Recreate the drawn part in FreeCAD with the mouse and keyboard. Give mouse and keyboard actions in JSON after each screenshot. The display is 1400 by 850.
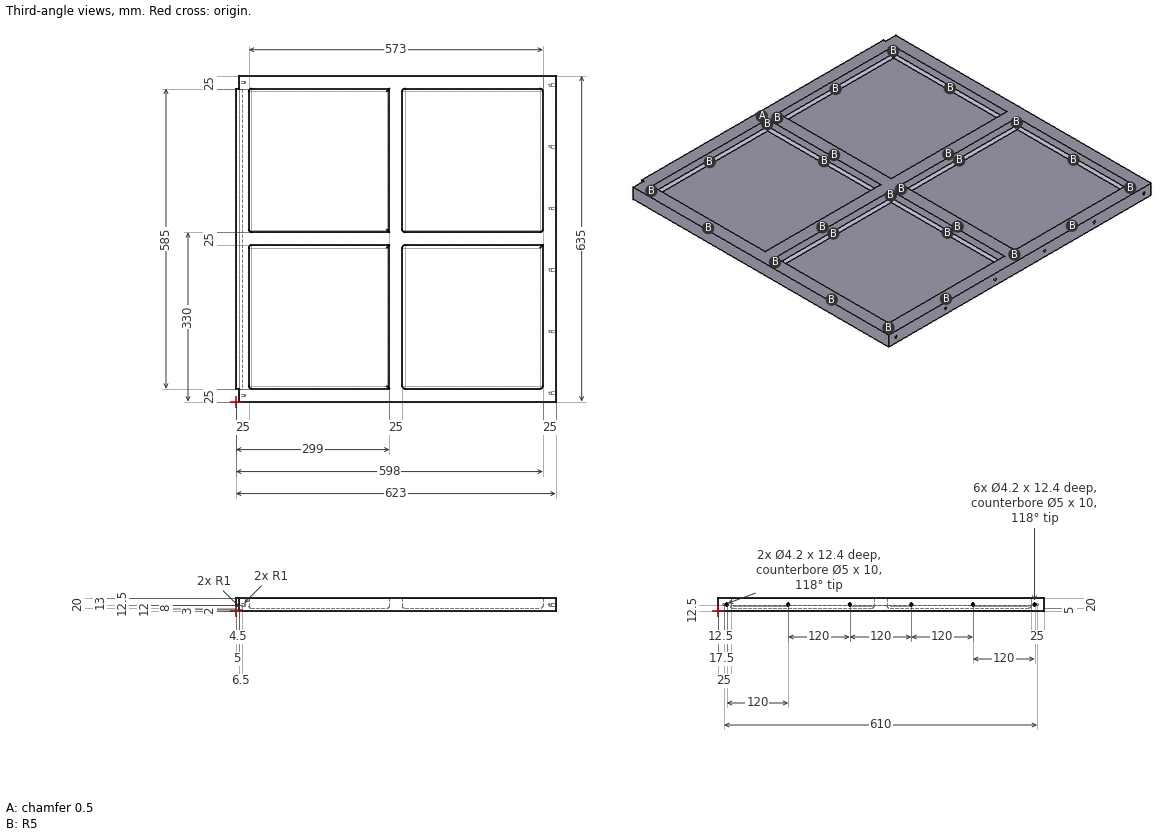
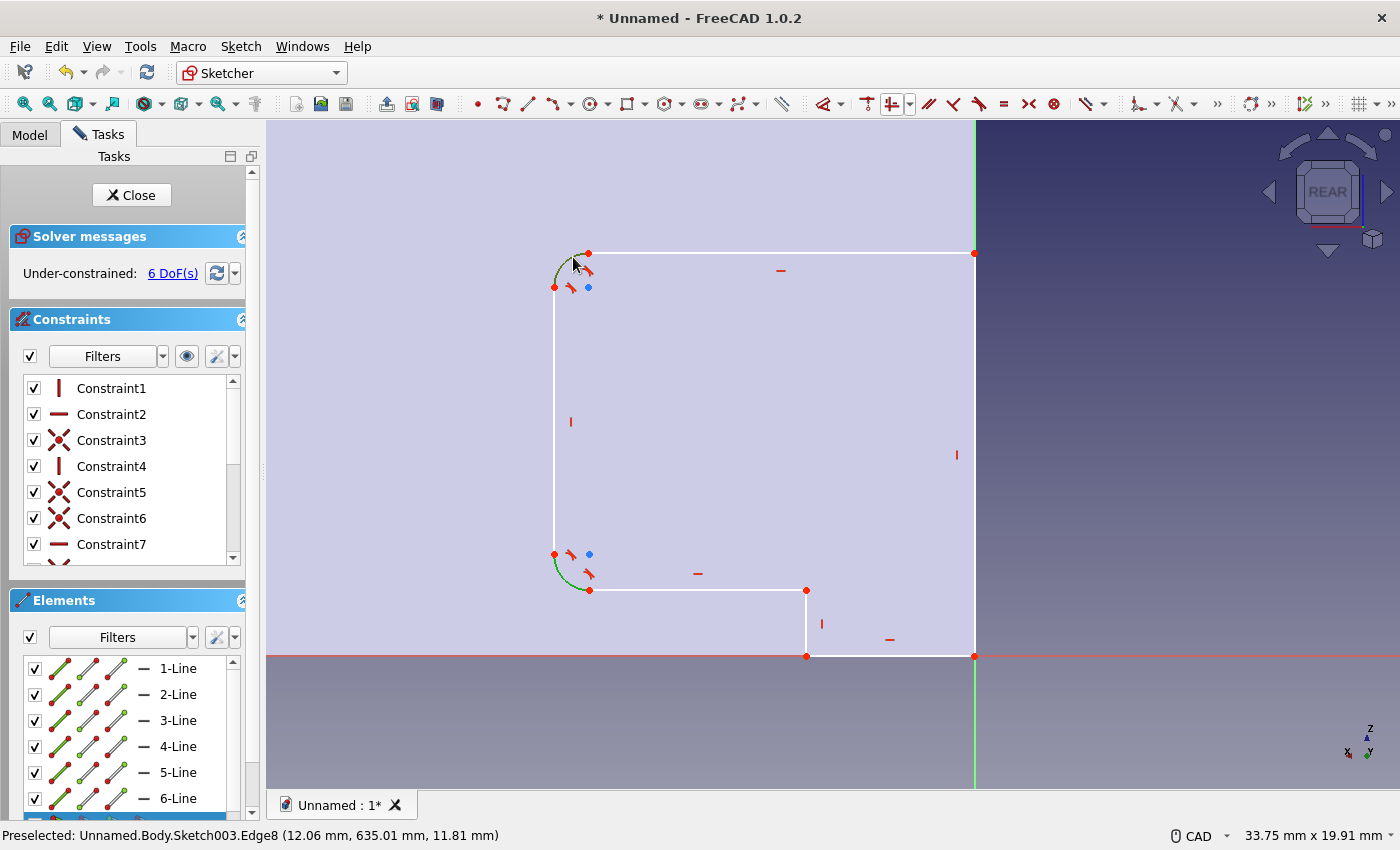
{"action": "left_click", "coordinate": [1004, 104]}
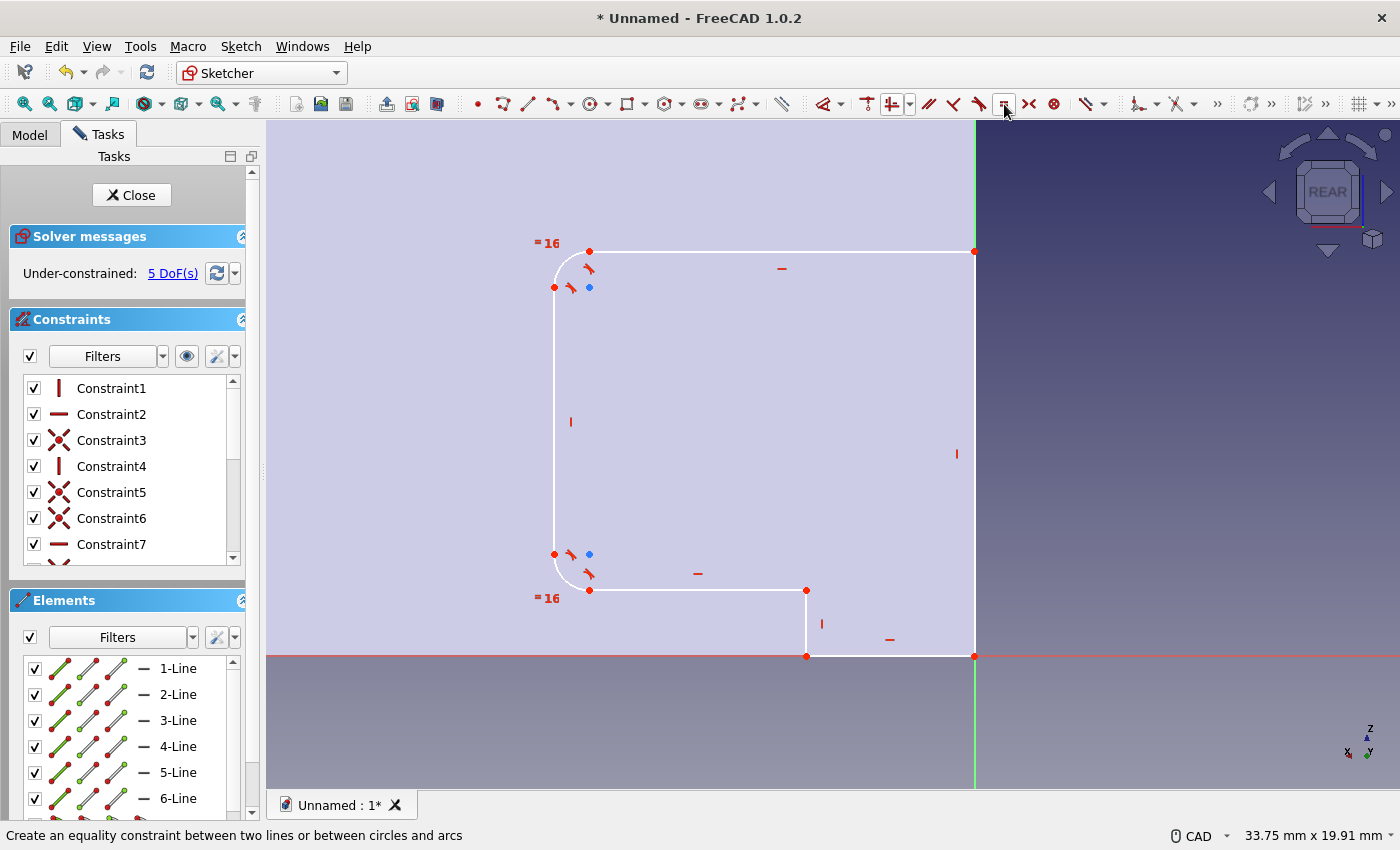
{"action": "left_click", "coordinate": [822, 104]}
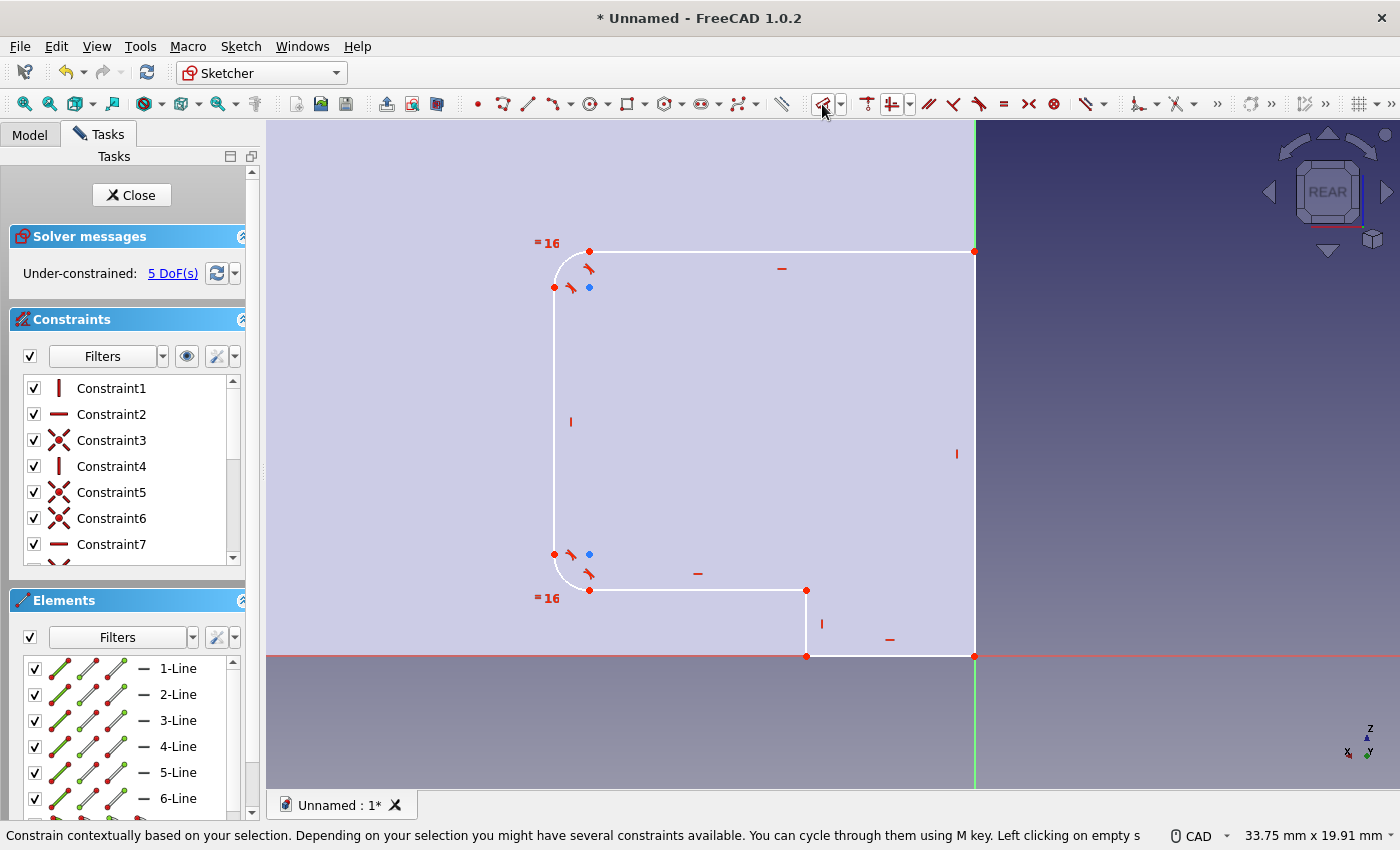
{"action": "left_click", "coordinate": [558, 571]}
{"action": "left_click", "coordinate": [529, 586]}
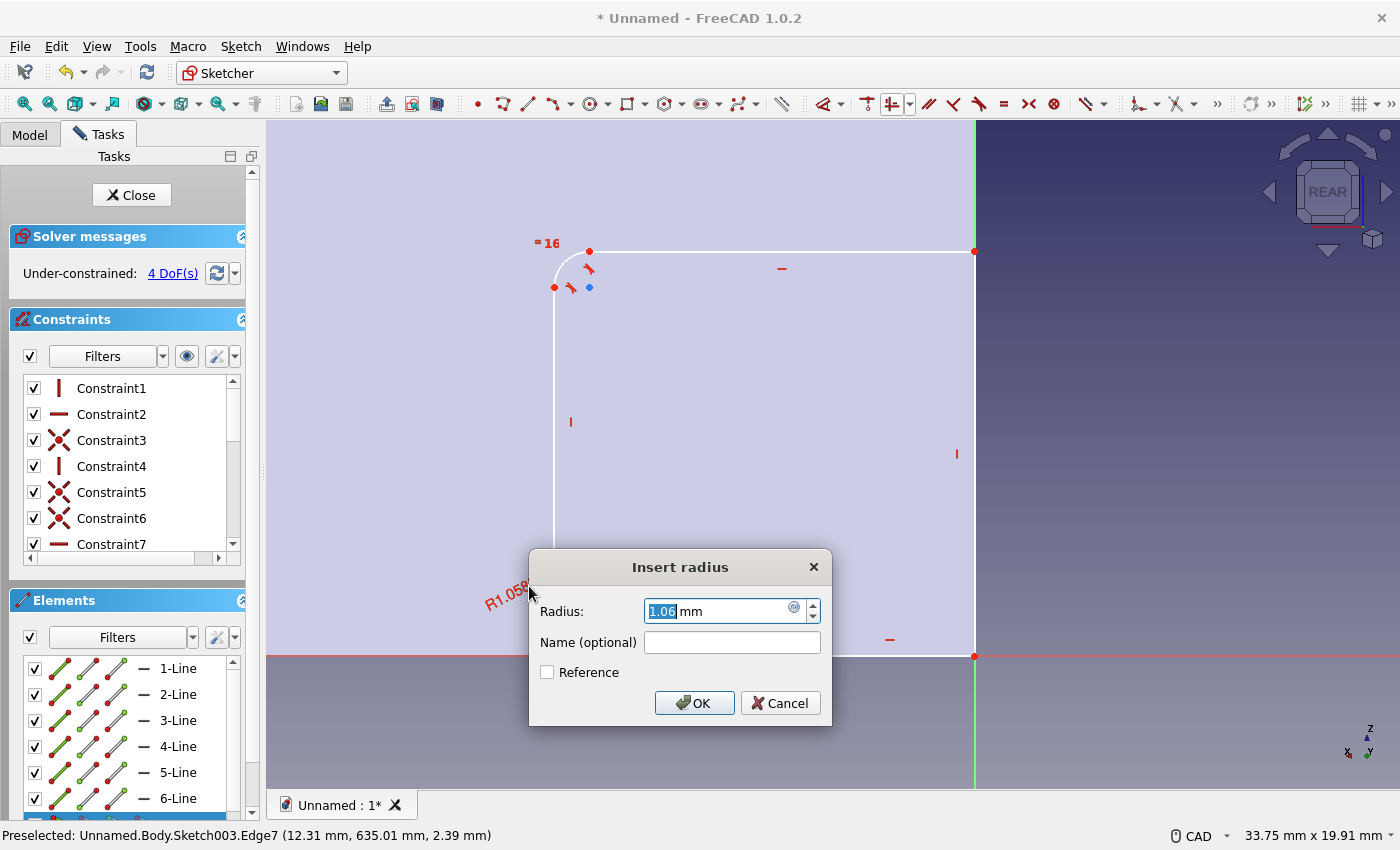
{"action": "type", "text": "1"}
{"action": "key", "text": "Return"}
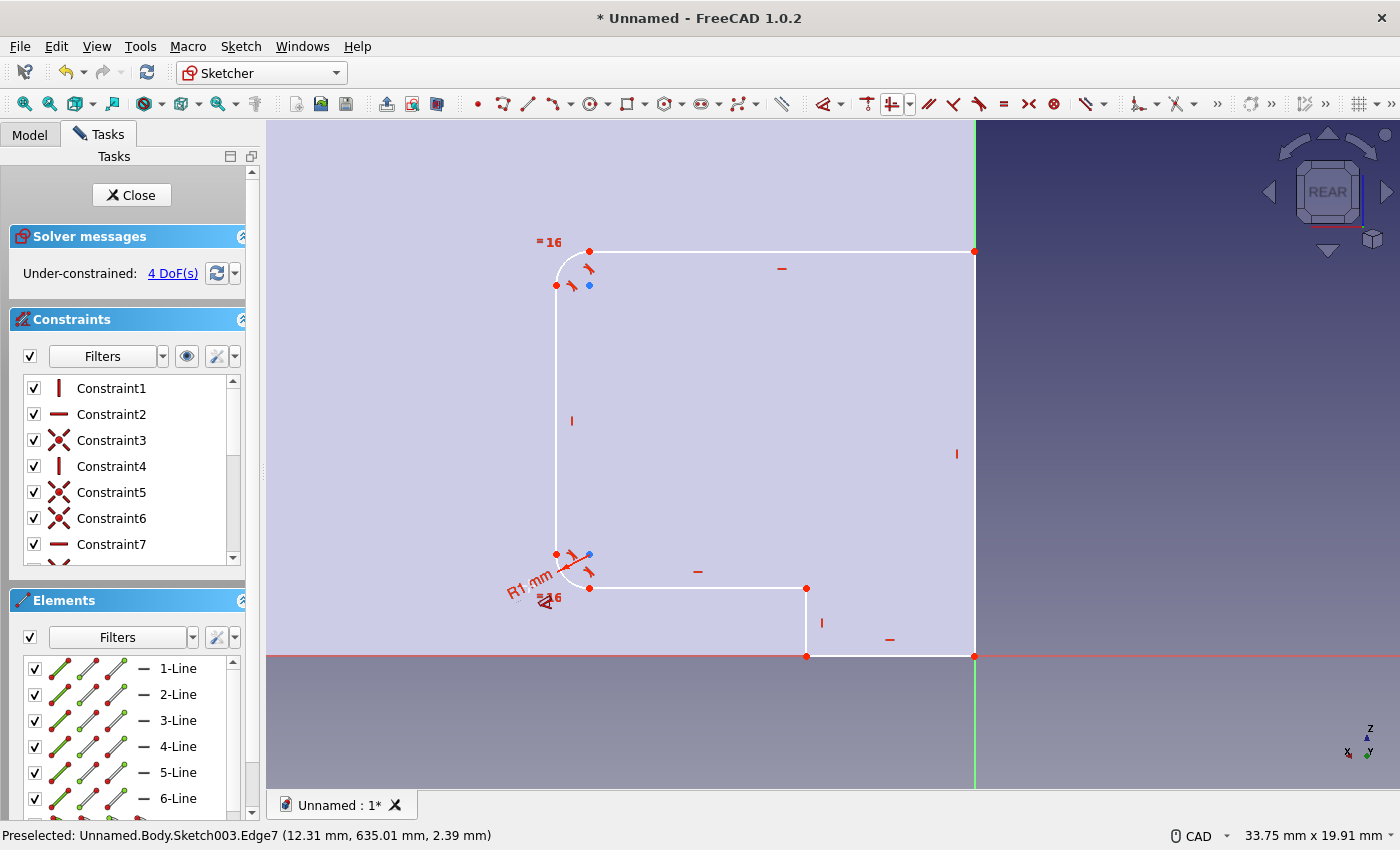
{"action": "left_click", "coordinate": [556, 366]}
{"action": "left_click", "coordinate": [522, 420]}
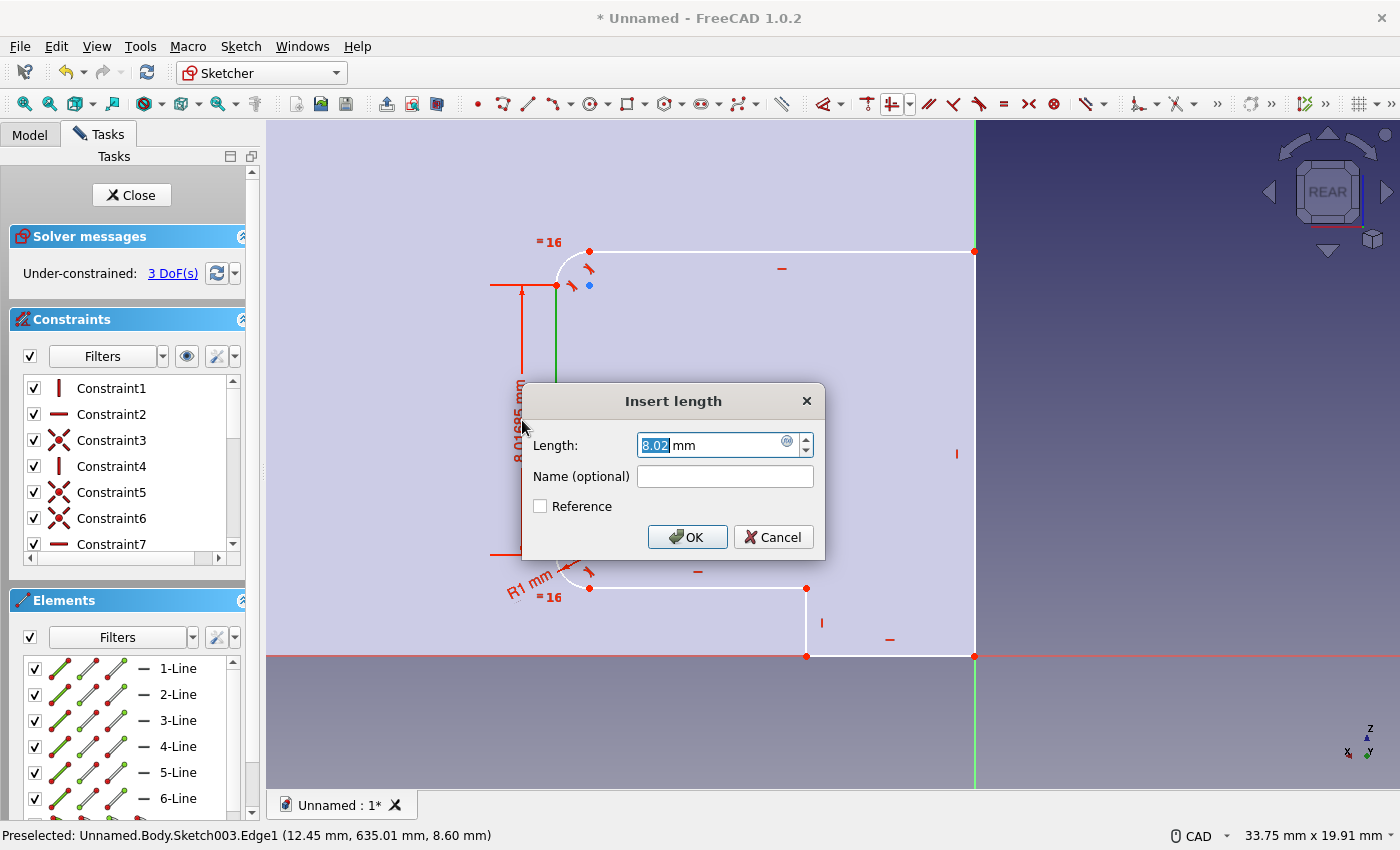
{"action": "type", "text": "8"}
{"action": "key", "text": "Return"}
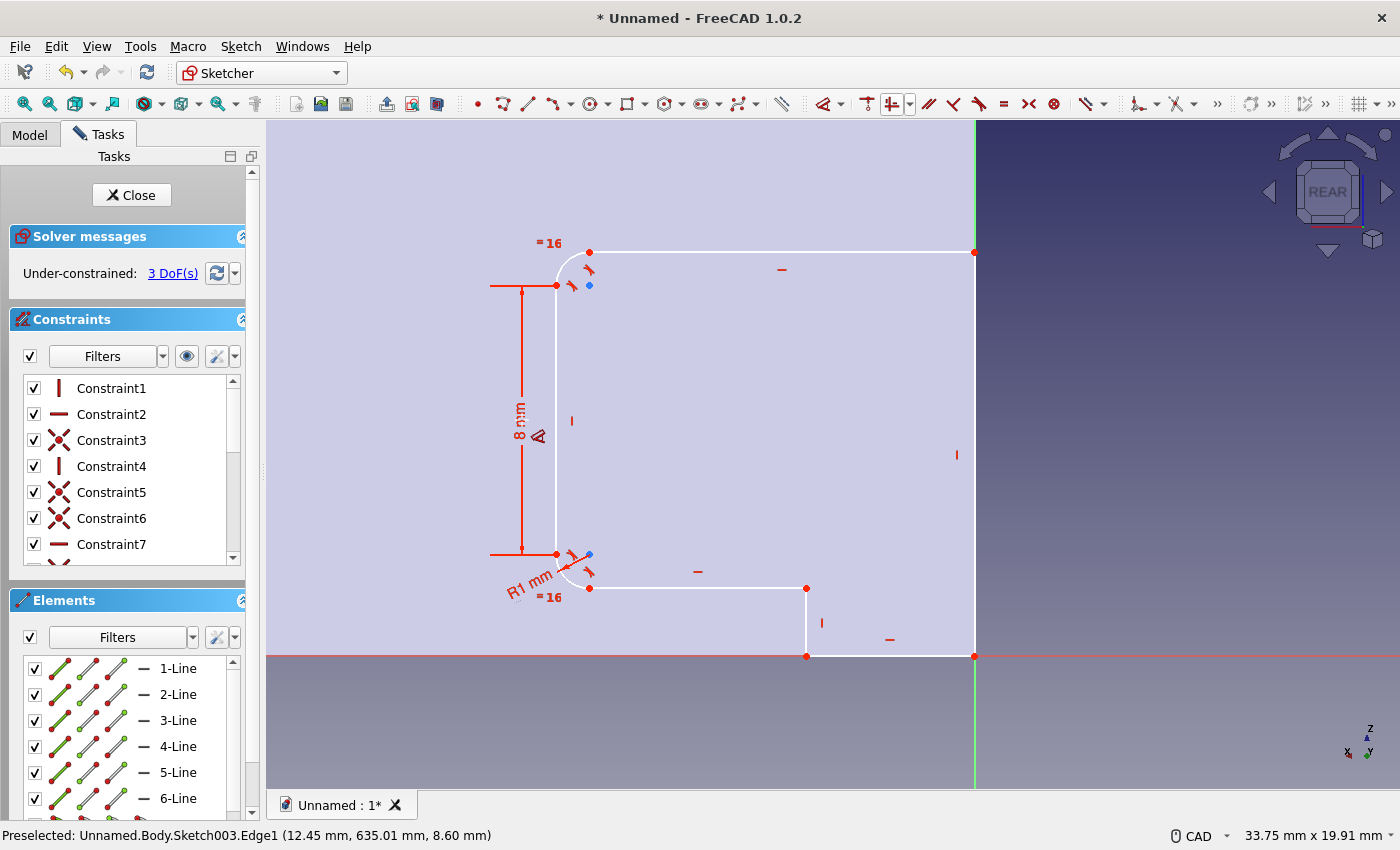
{"action": "left_click", "coordinate": [806, 609]}
{"action": "left_click", "coordinate": [840, 622]}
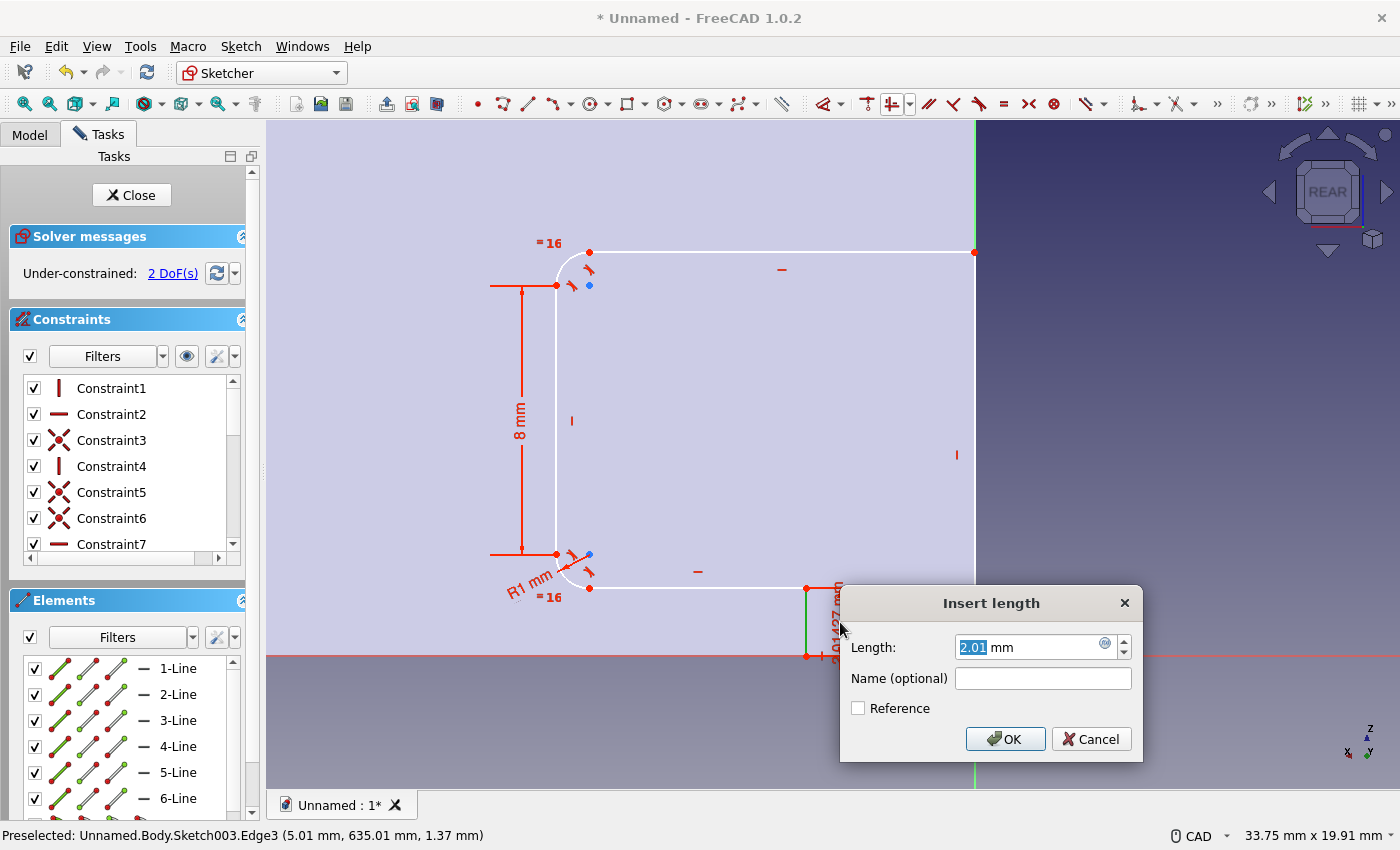
{"action": "type", "text": "2"}
{"action": "key", "text": "Return"}